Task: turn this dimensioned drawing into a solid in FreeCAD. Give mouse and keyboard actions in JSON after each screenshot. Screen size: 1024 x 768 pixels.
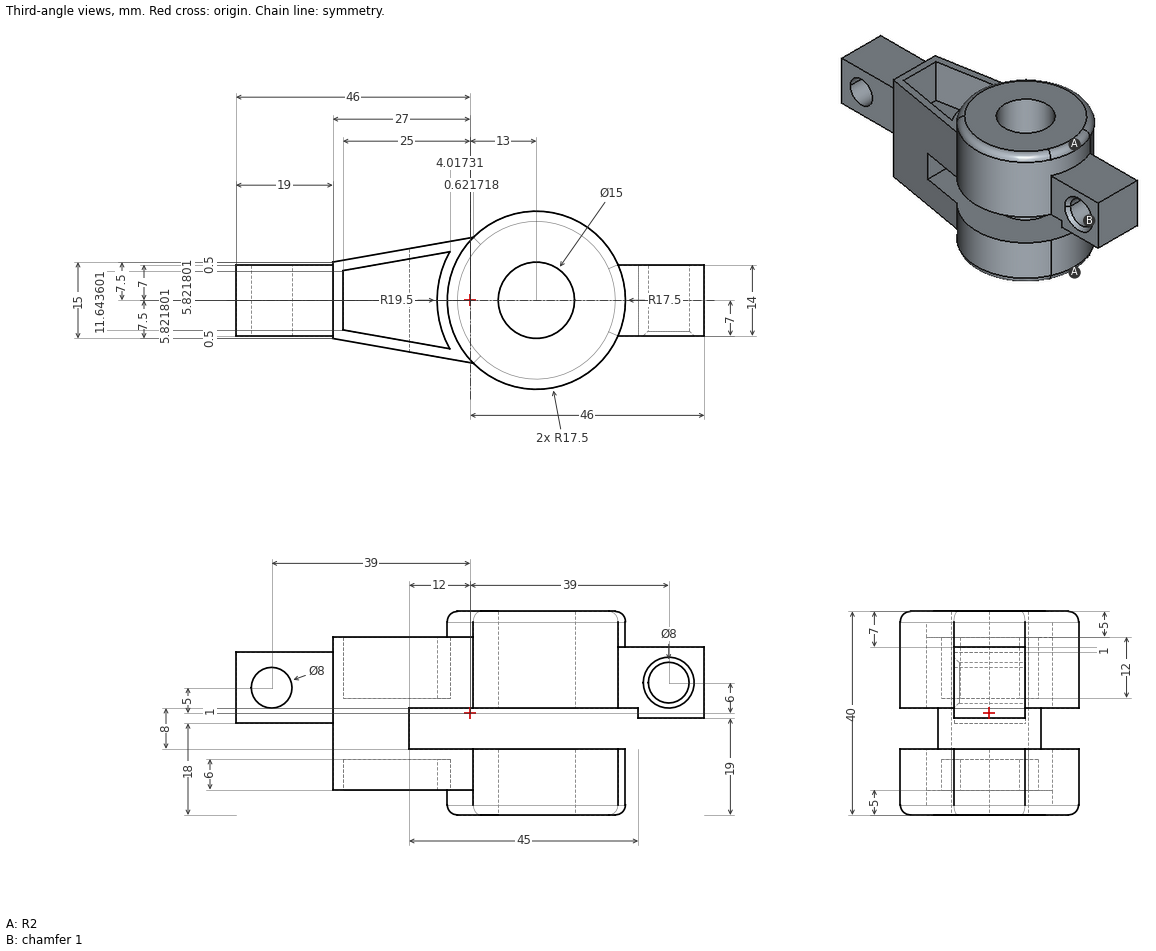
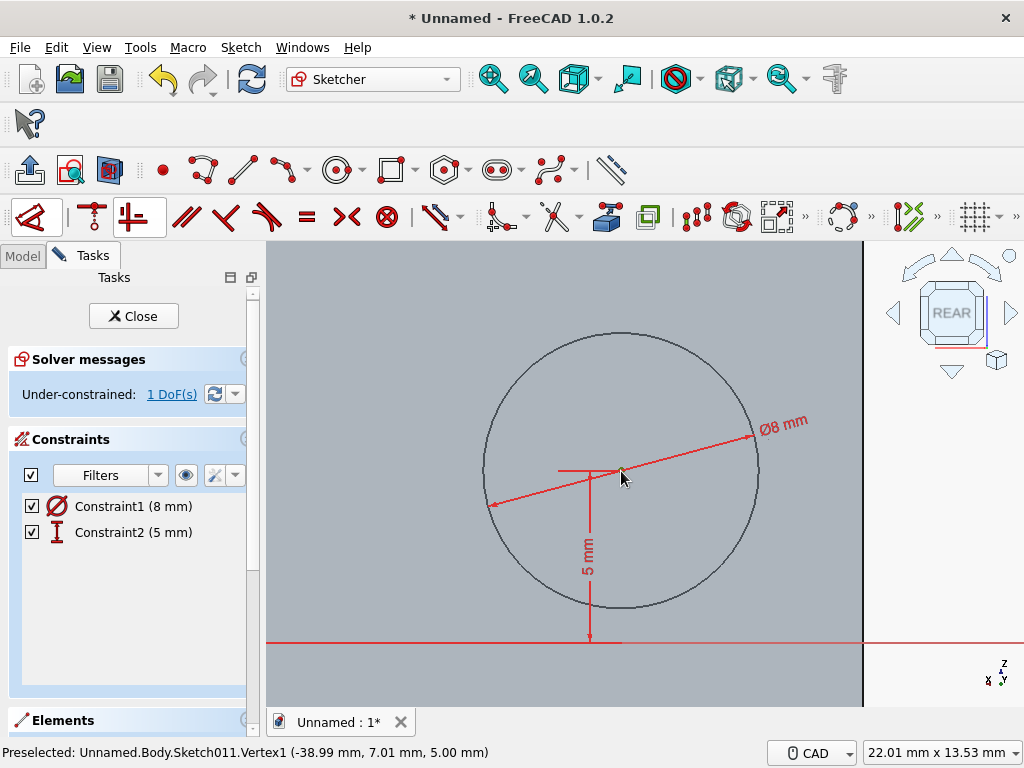
{"action": "left_click", "coordinate": [56, 218]}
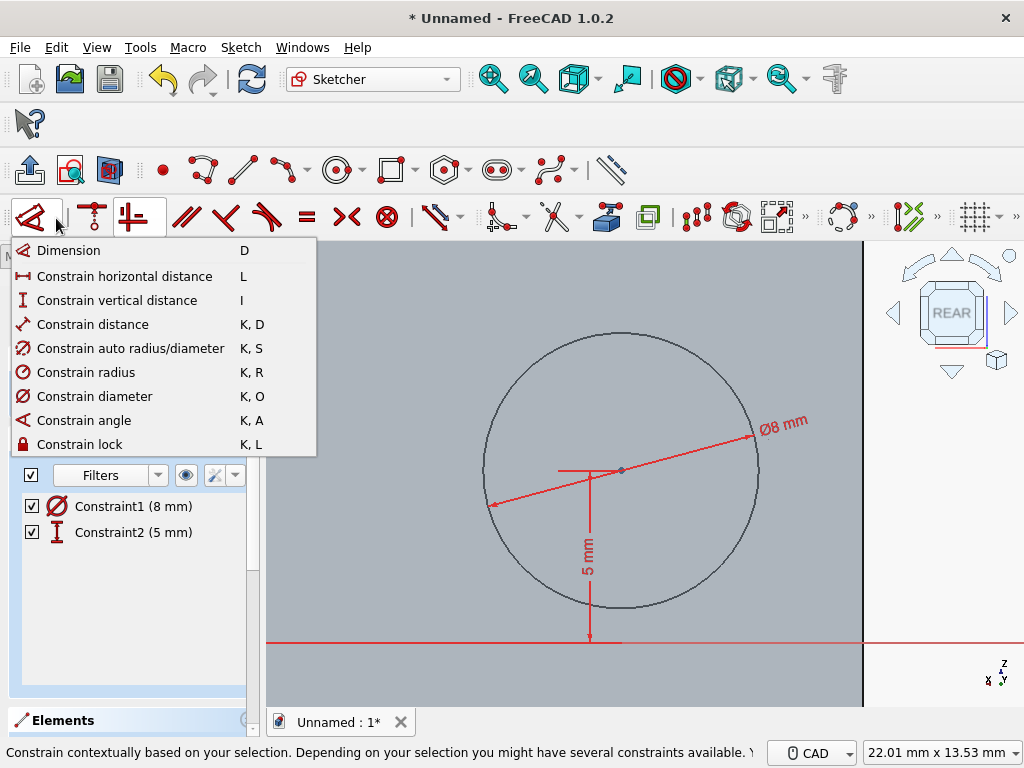
{"action": "left_click", "coordinate": [164, 276]}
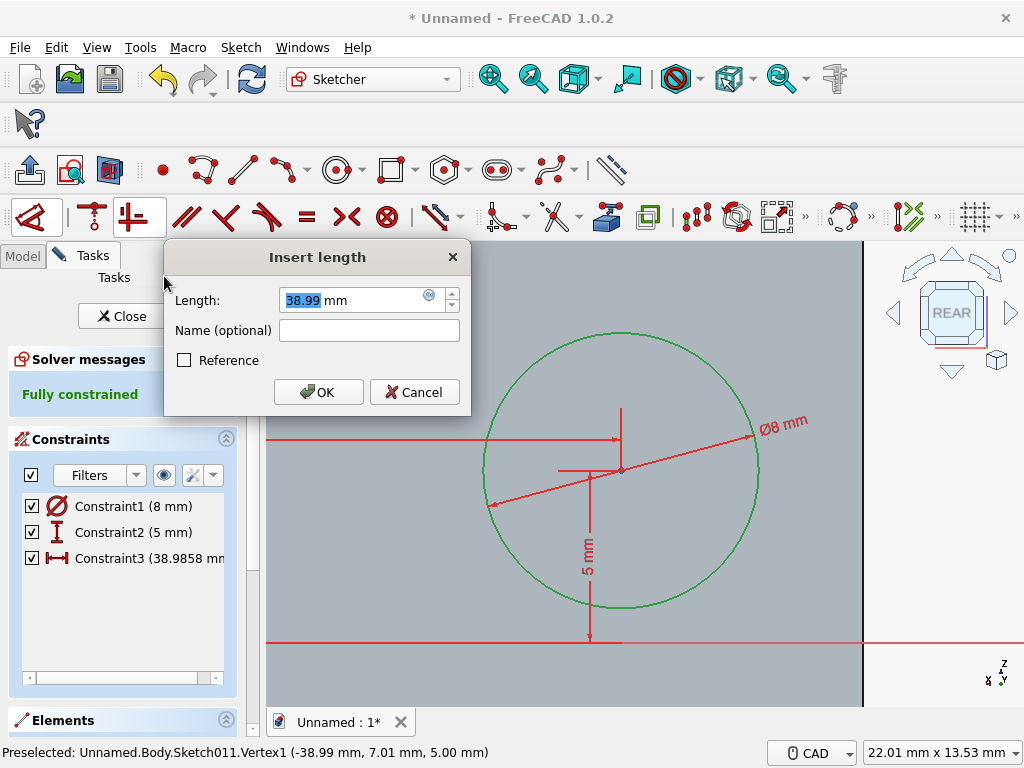
{"action": "type", "text": "39"}
{"action": "key", "text": "Return"}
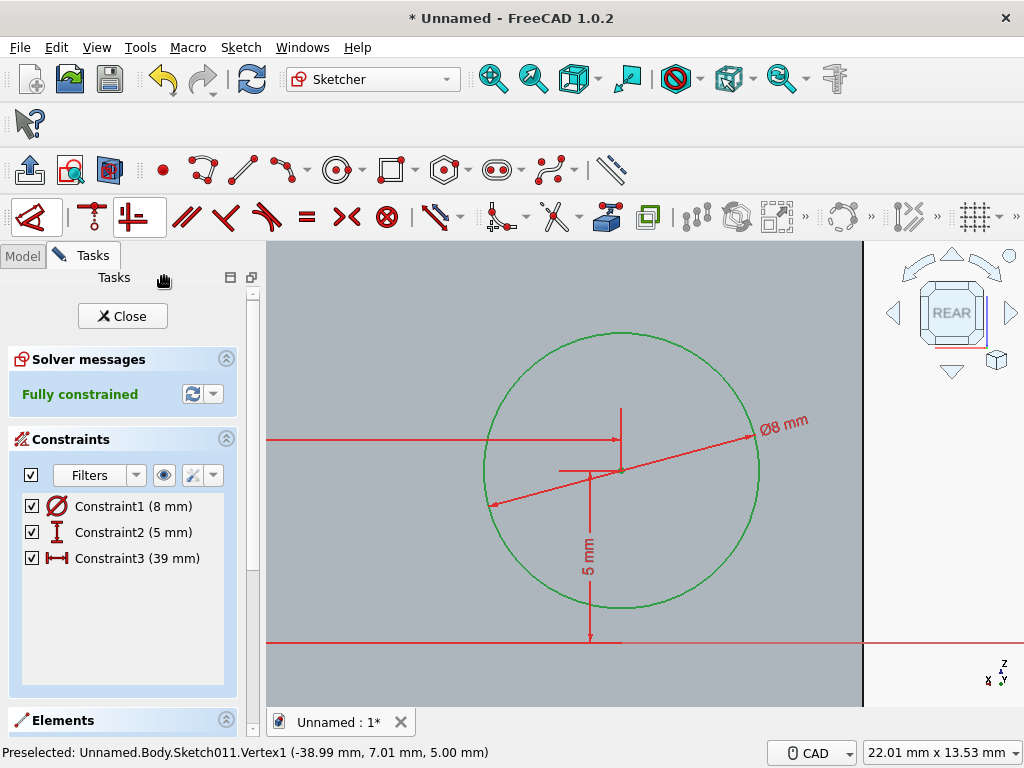
{"action": "left_click", "coordinate": [123, 316]}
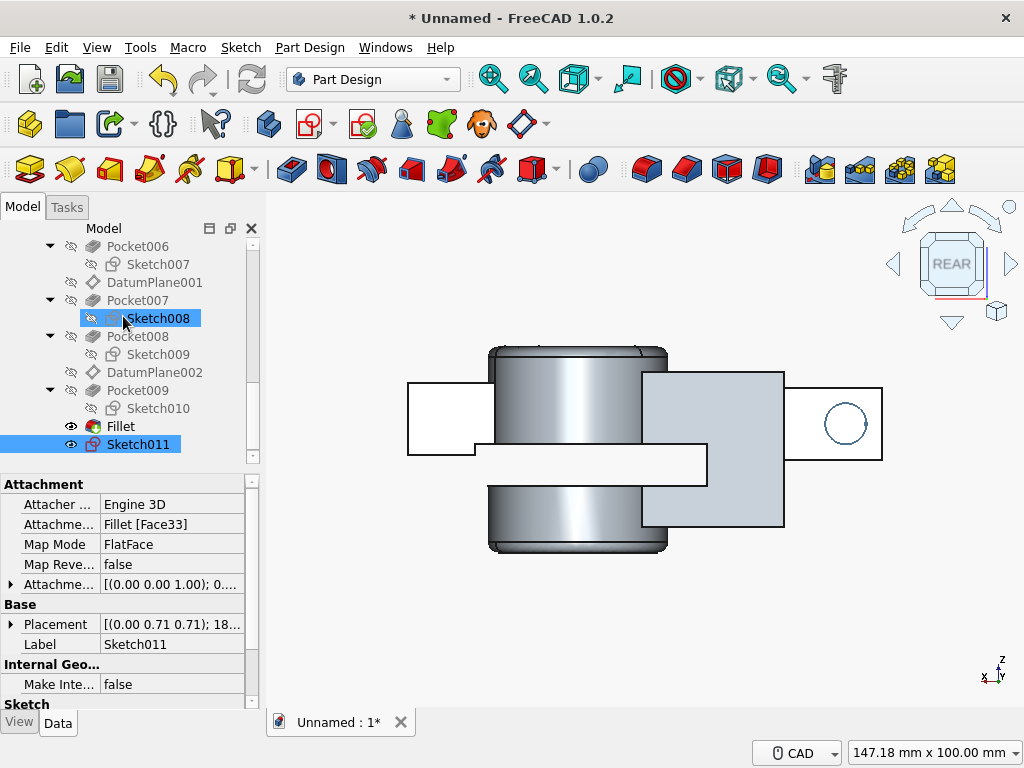
{"action": "left_click", "coordinate": [292, 170]}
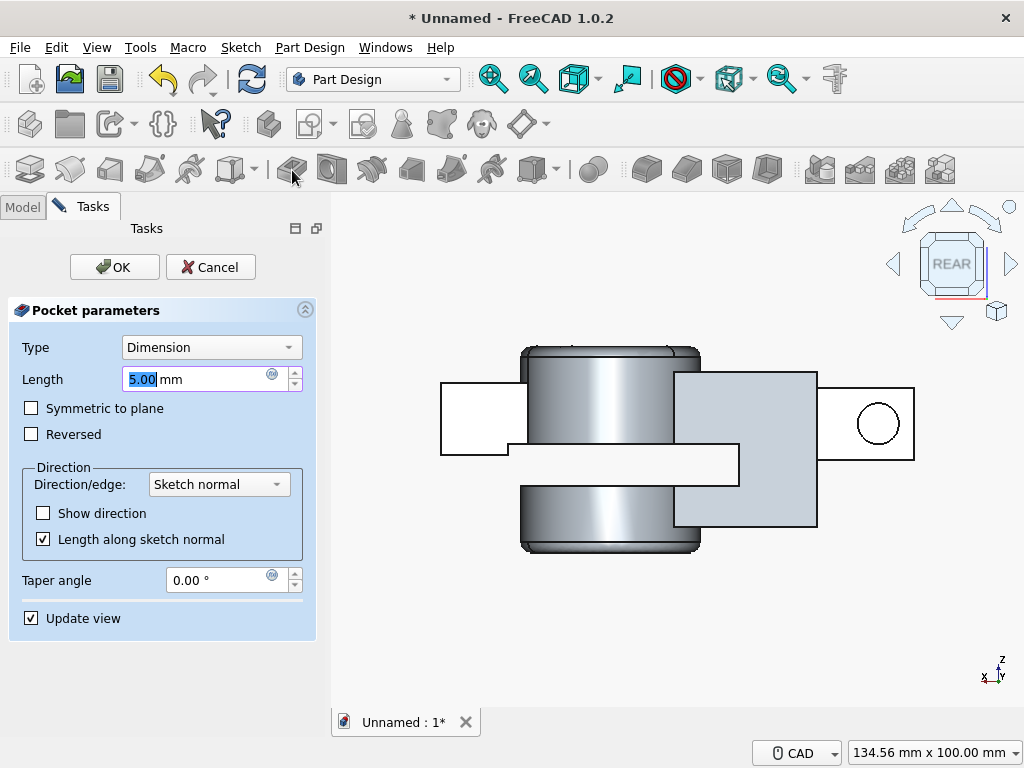
{"action": "left_click", "coordinate": [212, 348]}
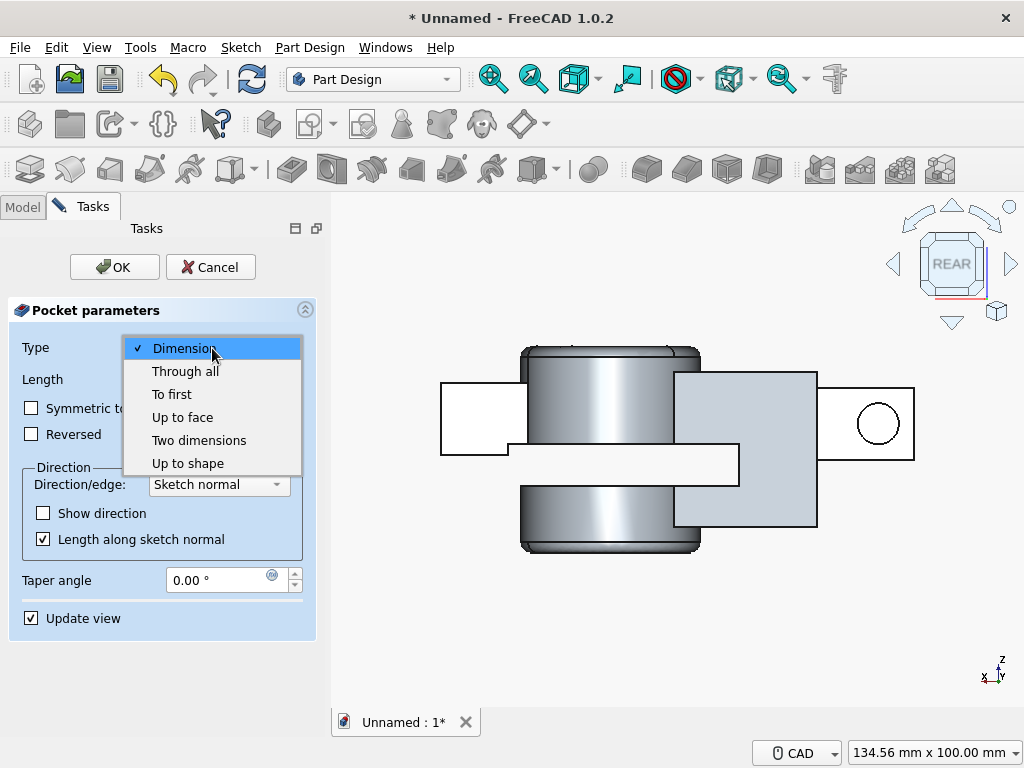
{"action": "left_click", "coordinate": [212, 394]}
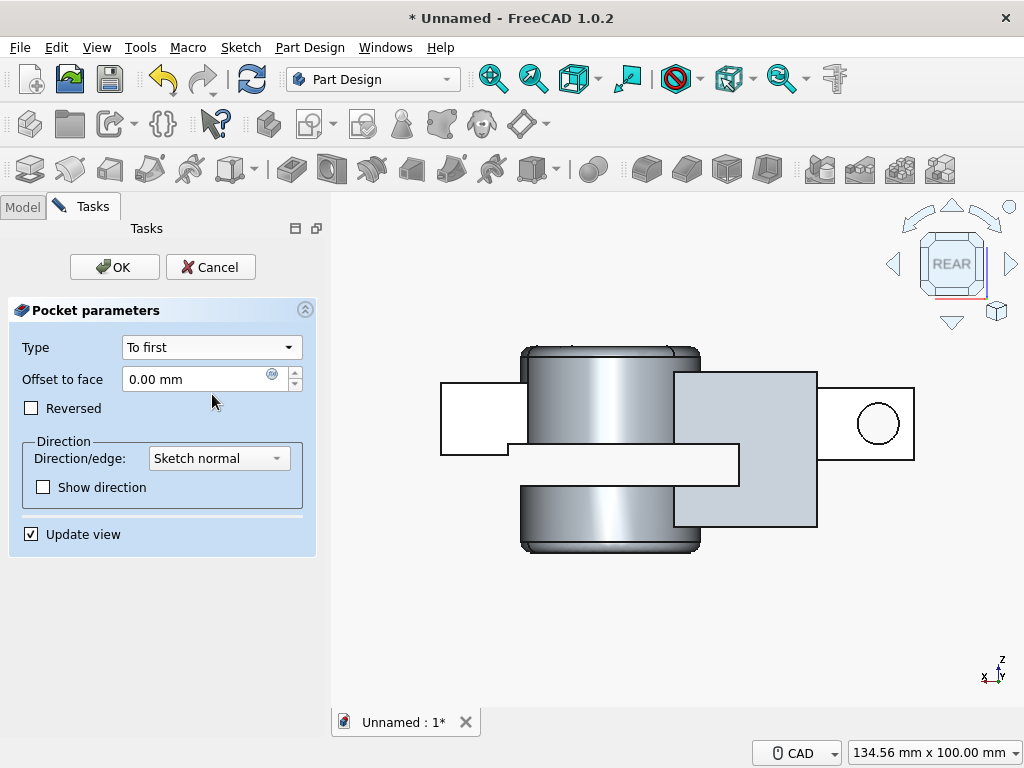
{"action": "left_click", "coordinate": [115, 267]}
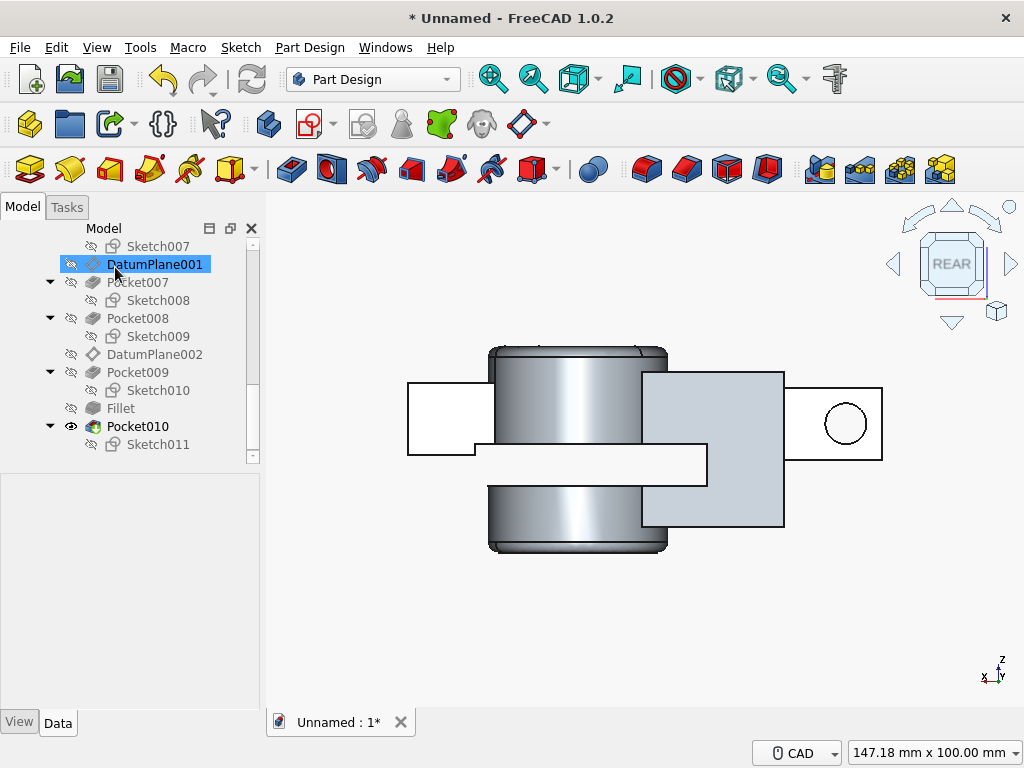
{"action": "left_click", "coordinate": [452, 418]}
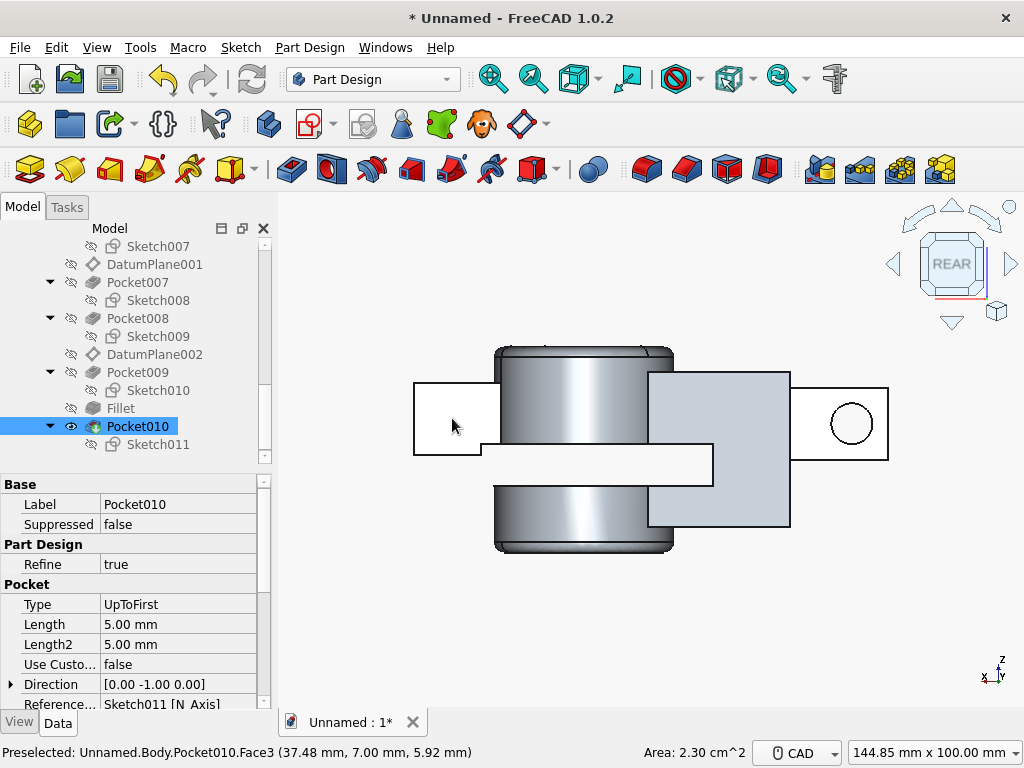
{"action": "left_click", "coordinate": [310, 124]}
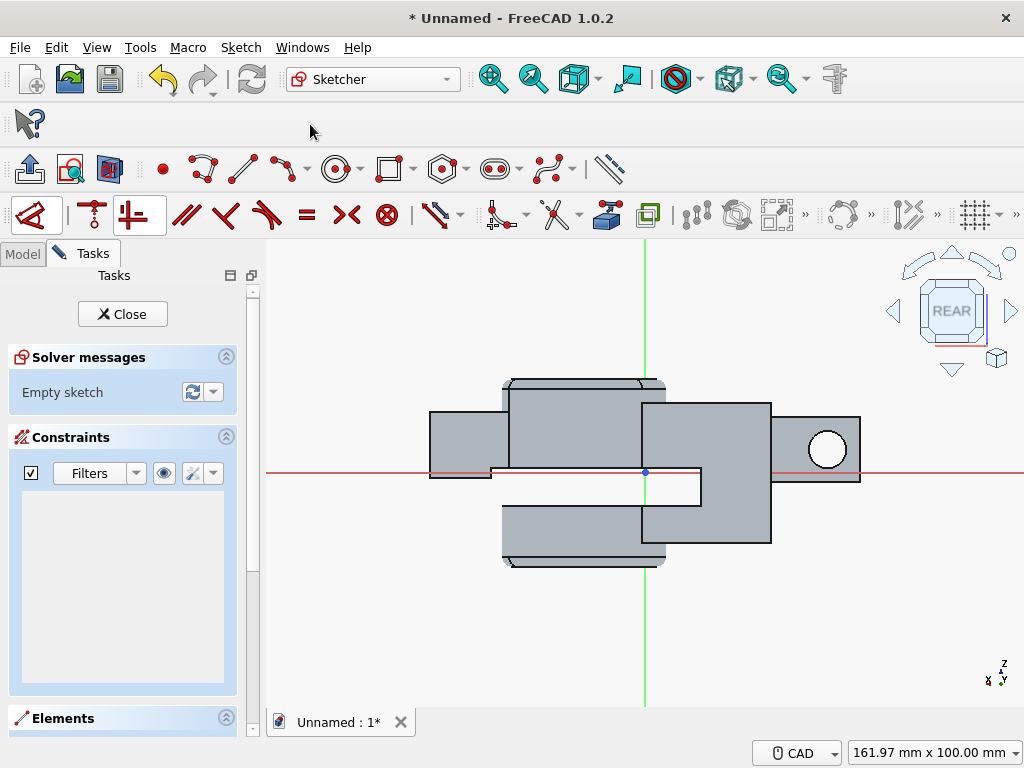
{"action": "scroll", "coordinate": [445, 441], "scroll_direction": "up", "scroll_amount": 10}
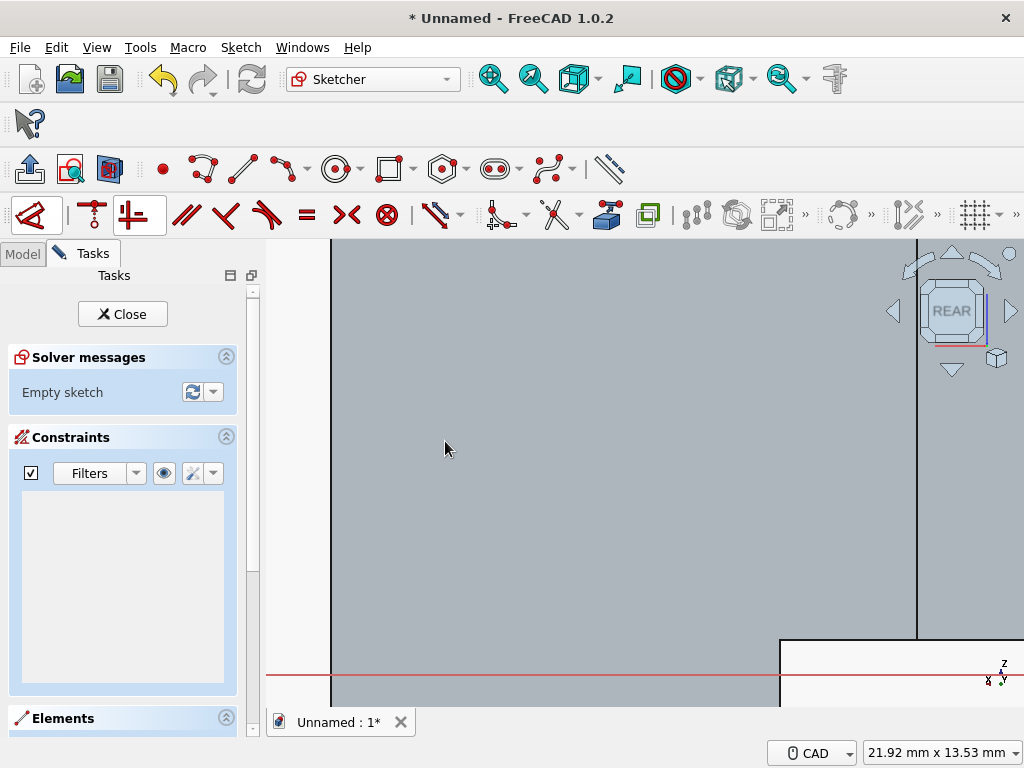
{"action": "left_click", "coordinate": [336, 170]}